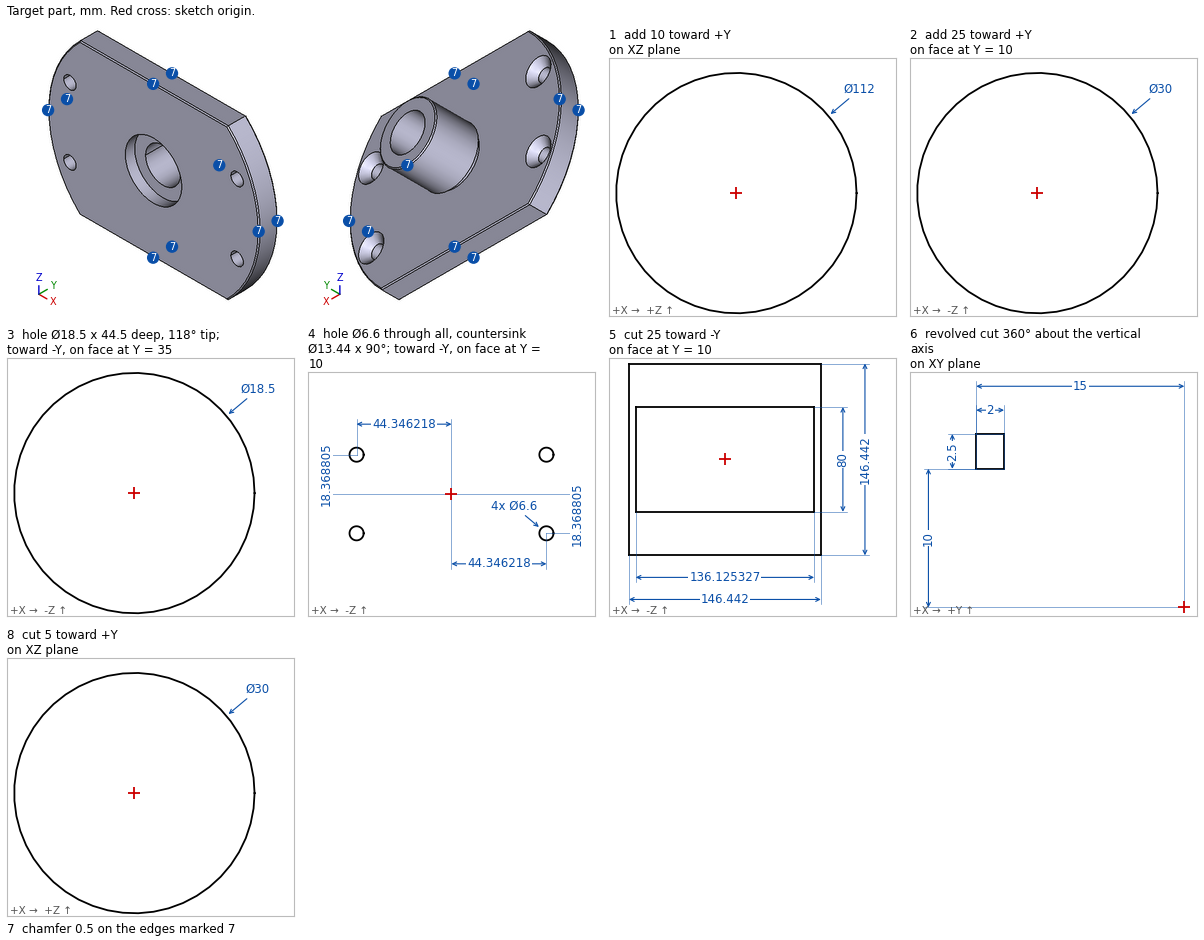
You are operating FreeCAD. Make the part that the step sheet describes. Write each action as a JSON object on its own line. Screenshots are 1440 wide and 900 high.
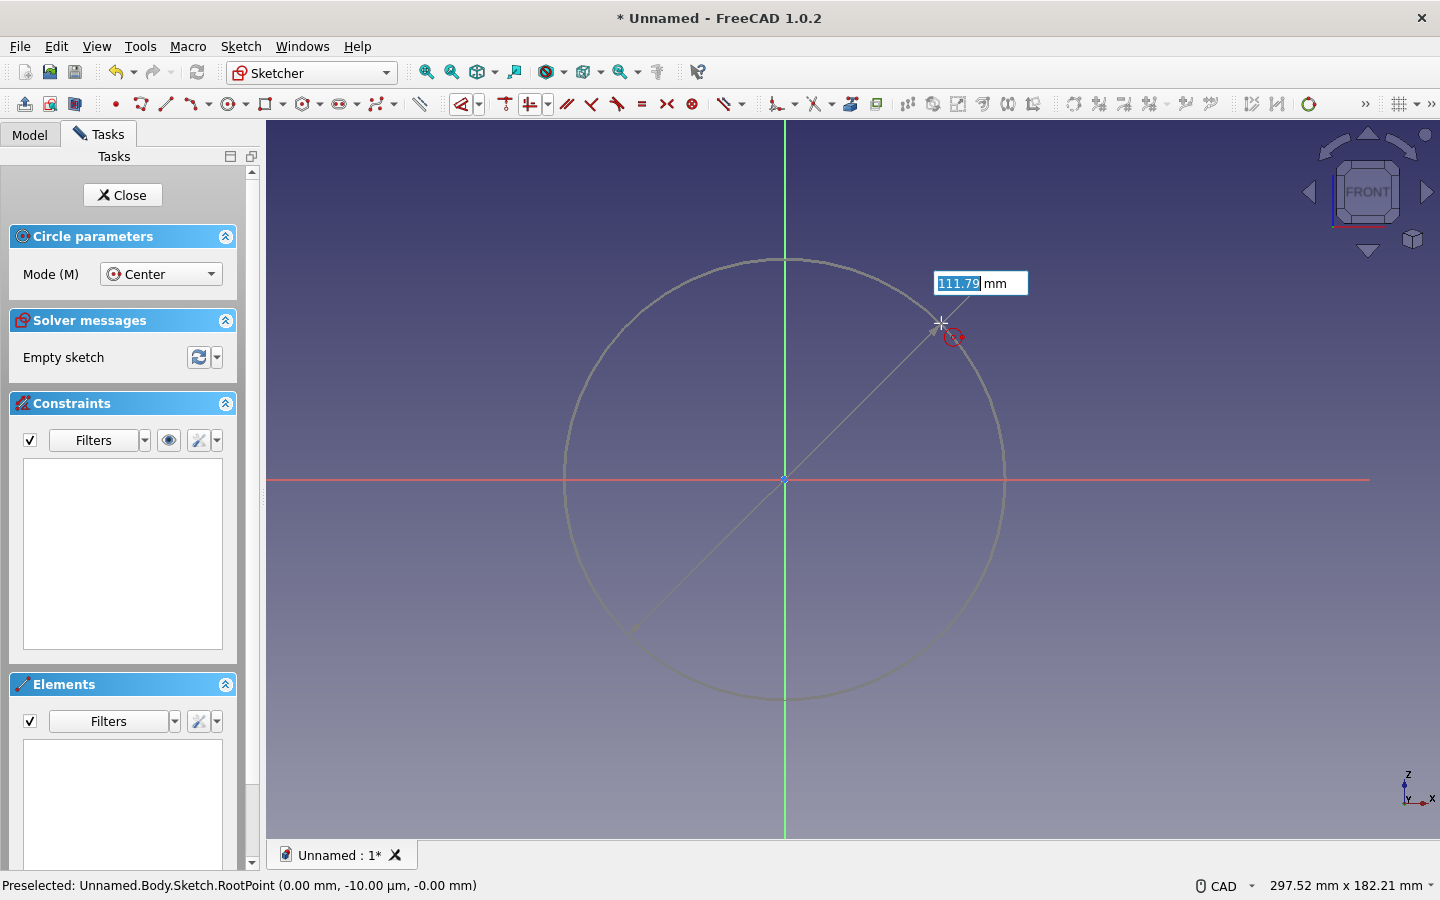
{"action": "type", "text": "112"}
{"action": "key", "text": "Return"}
{"action": "key", "text": "Escape"}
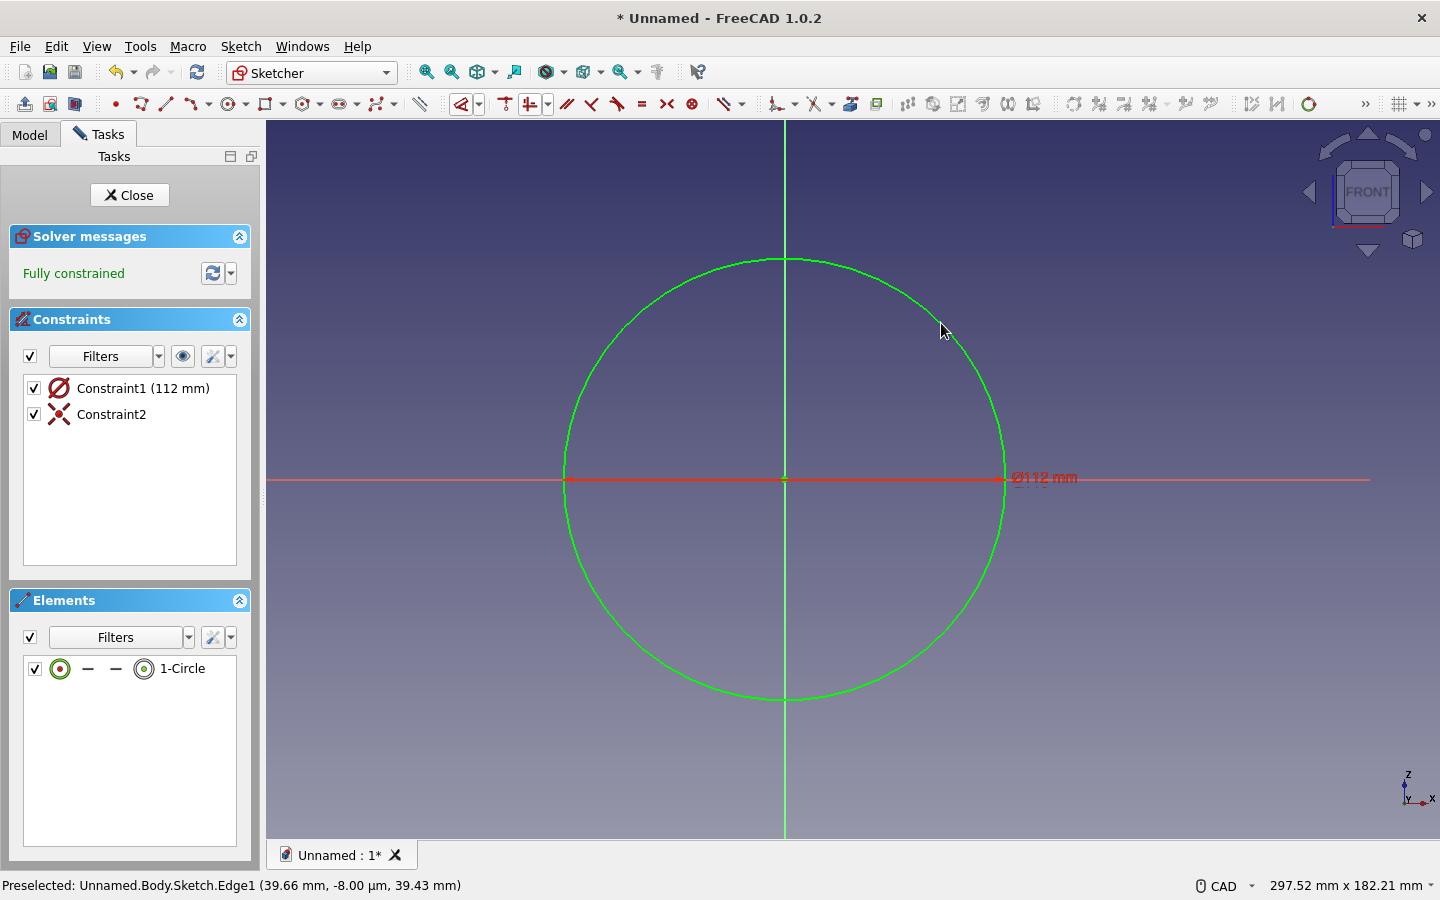
{"action": "left_click", "coordinate": [130, 195]}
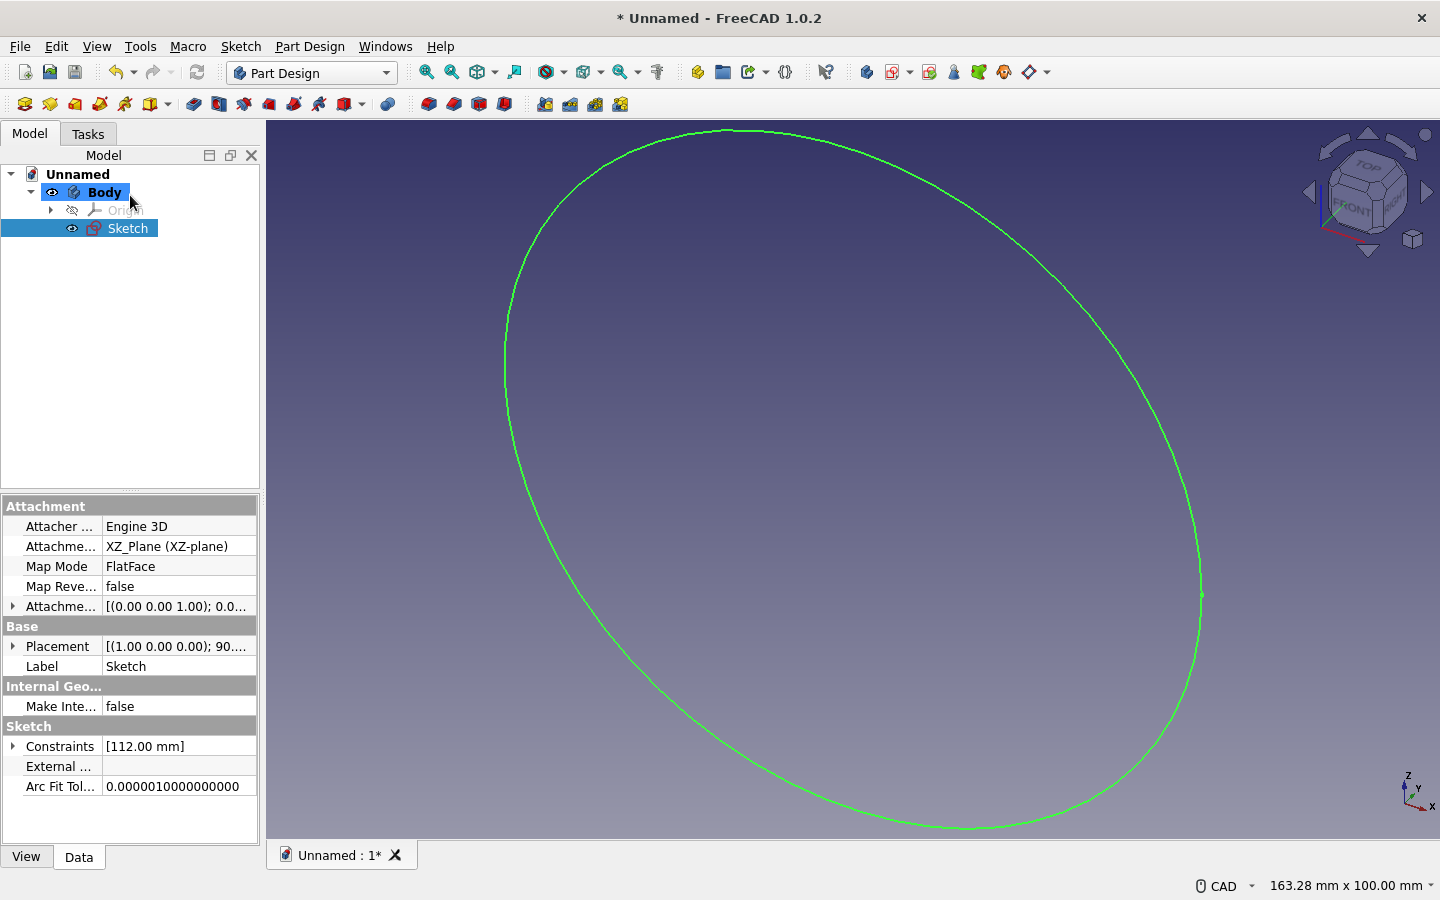
{"action": "left_click", "coordinate": [25, 104]}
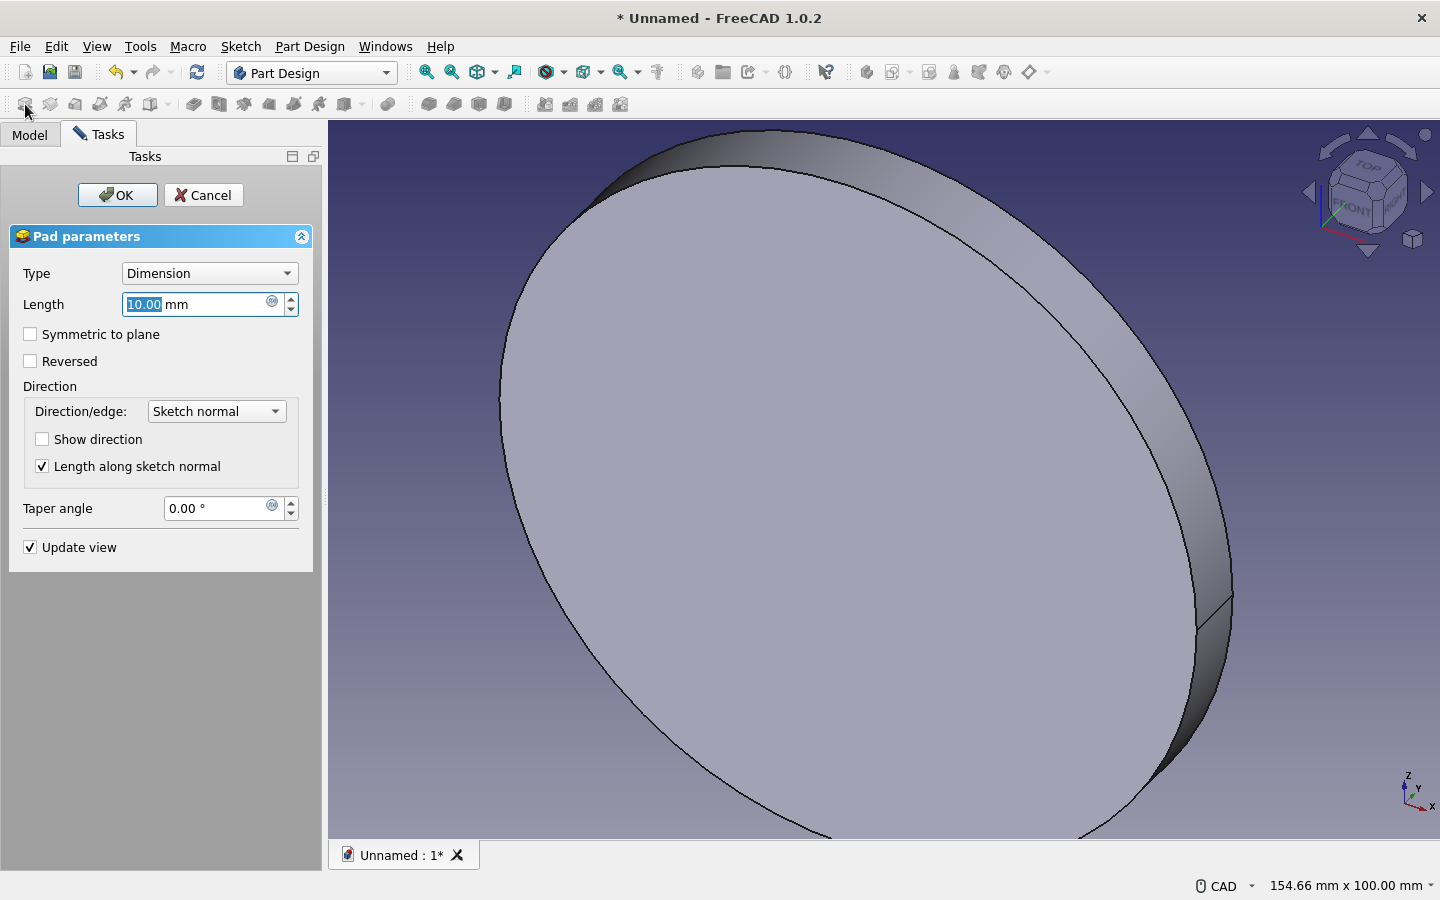
{"action": "type", "text": "10"}
{"action": "key", "text": "Tab"}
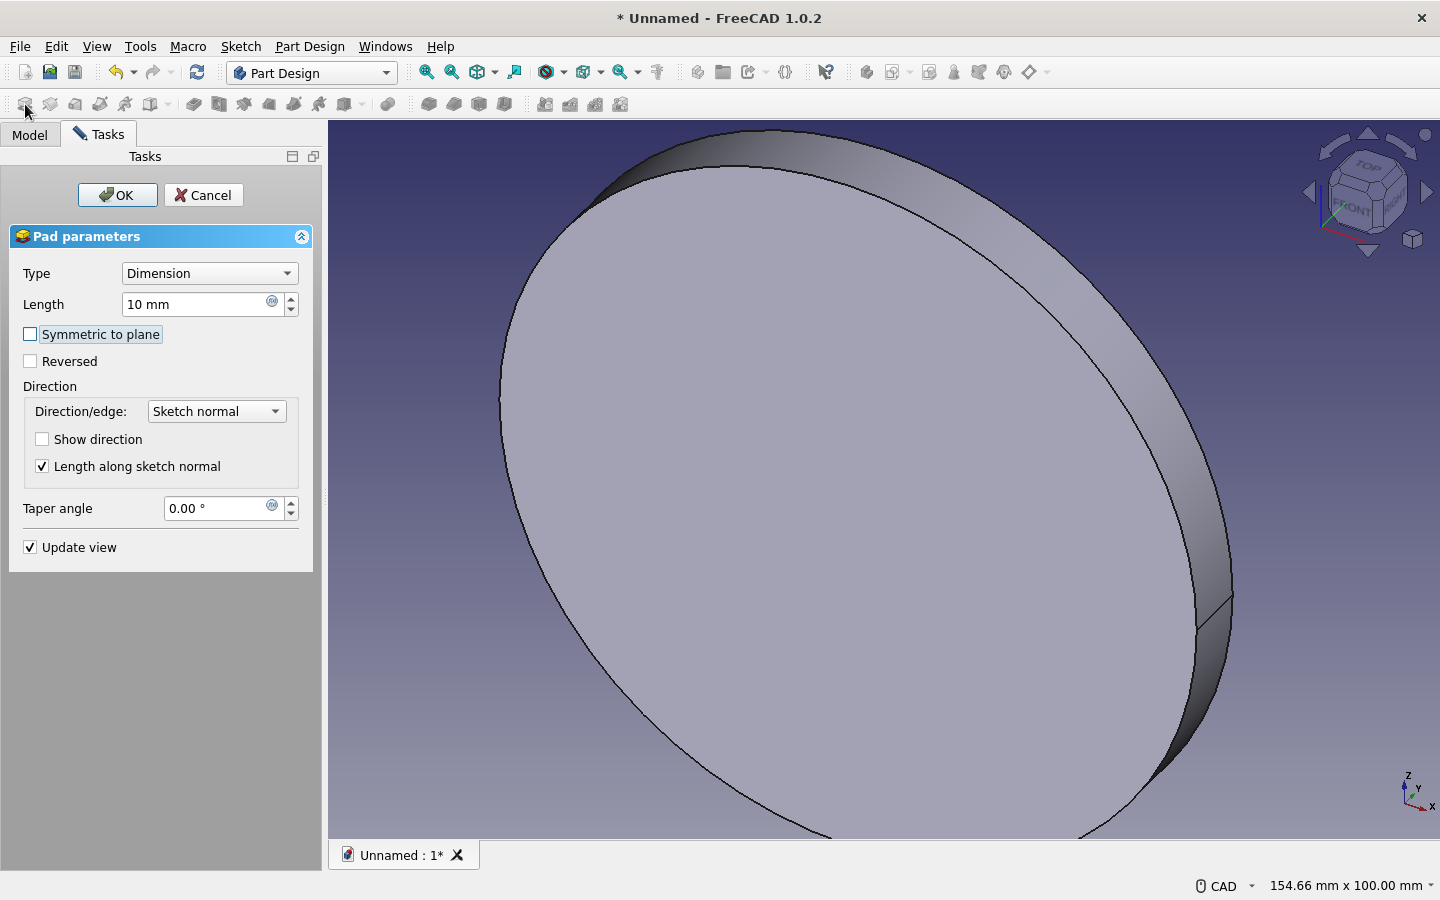
{"action": "left_click", "coordinate": [31, 361]}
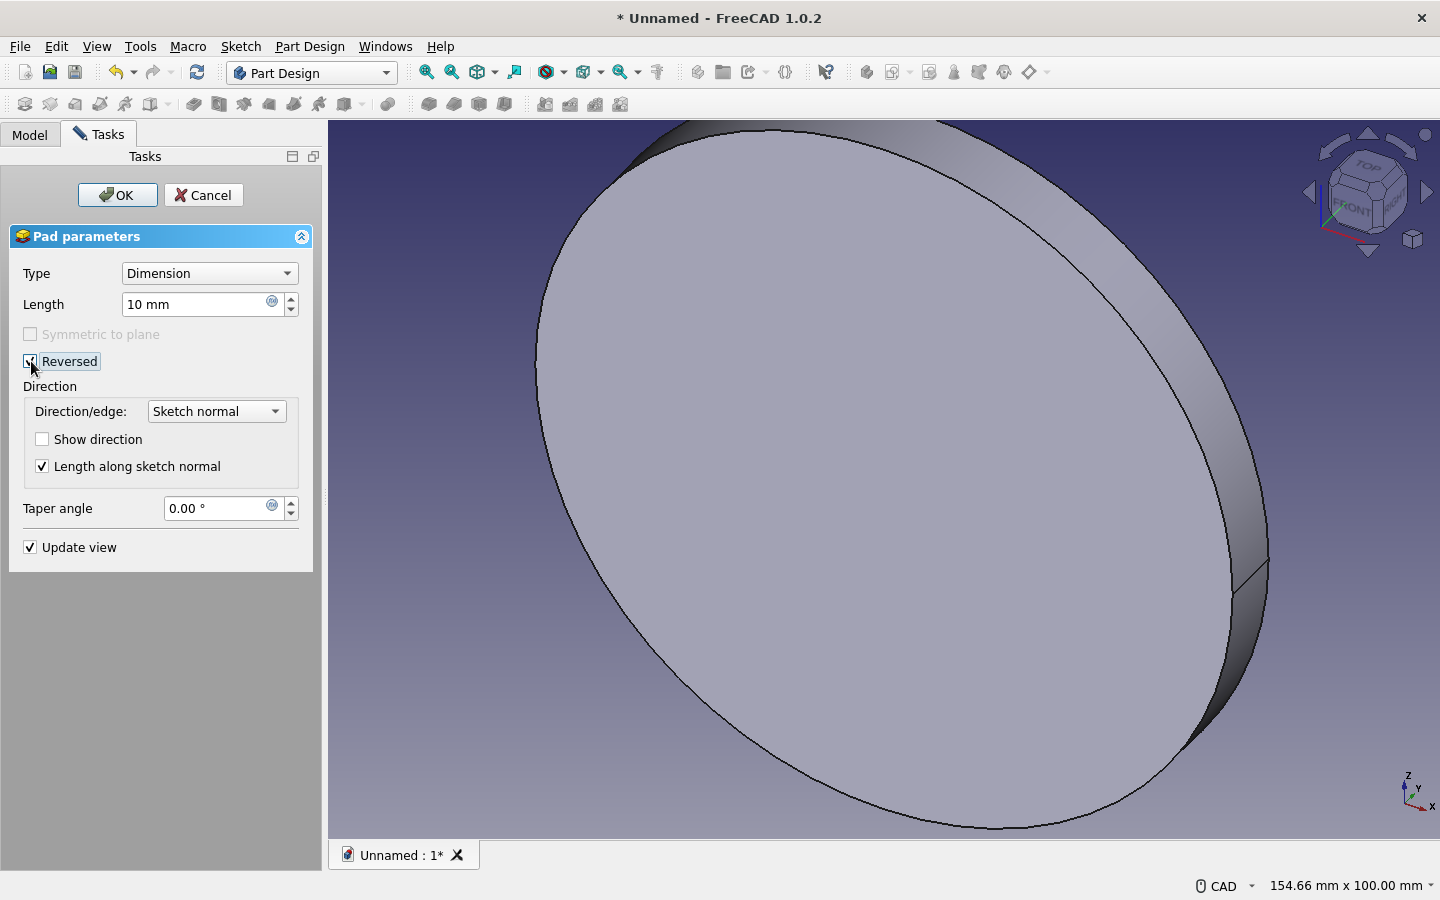
{"action": "left_click", "coordinate": [118, 195]}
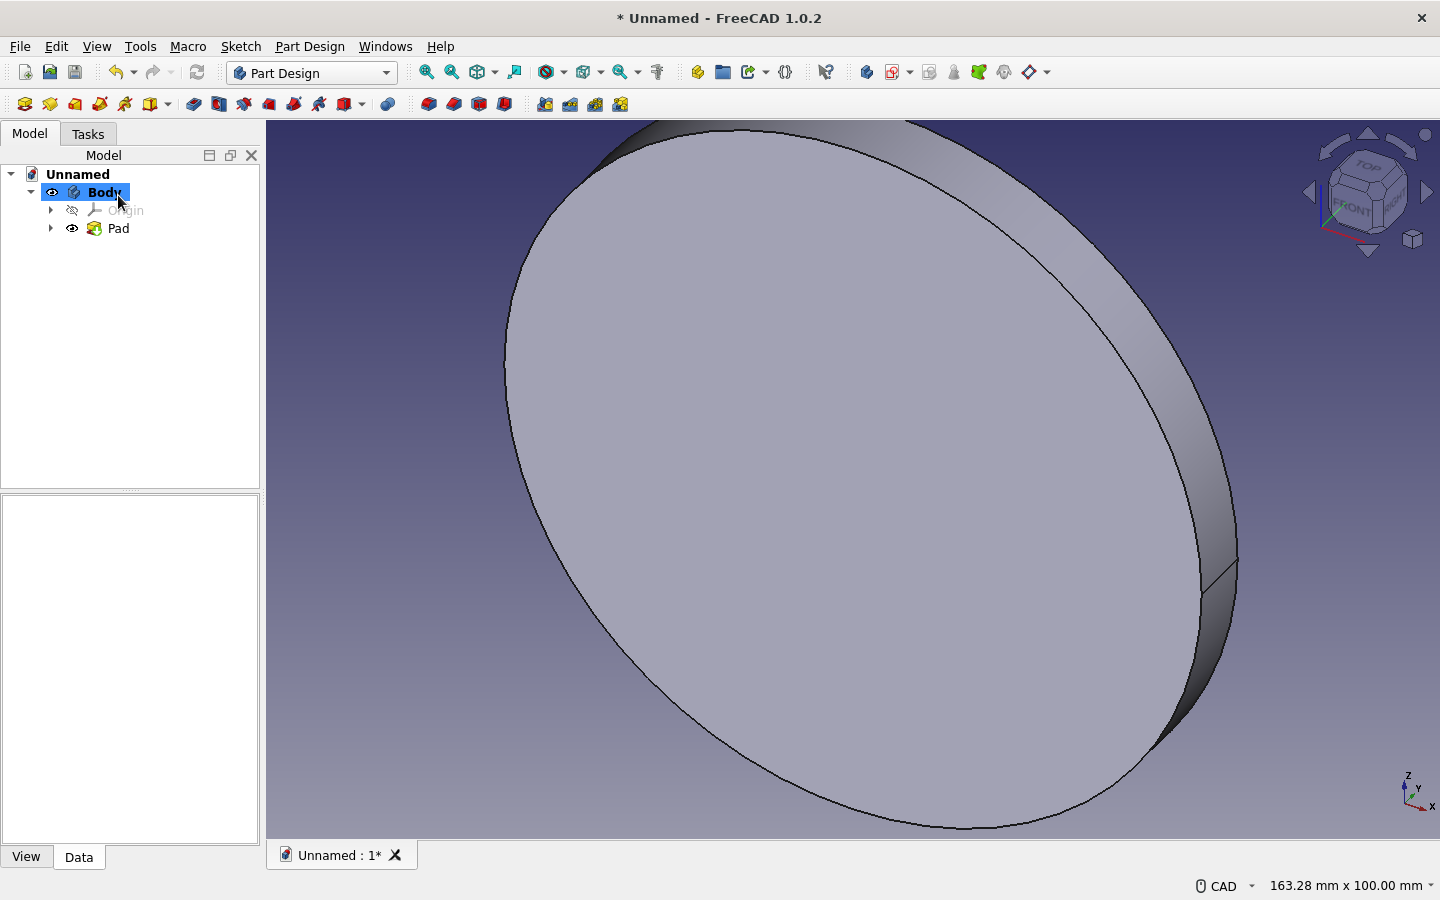
{"action": "left_click", "coordinate": [427, 72]}